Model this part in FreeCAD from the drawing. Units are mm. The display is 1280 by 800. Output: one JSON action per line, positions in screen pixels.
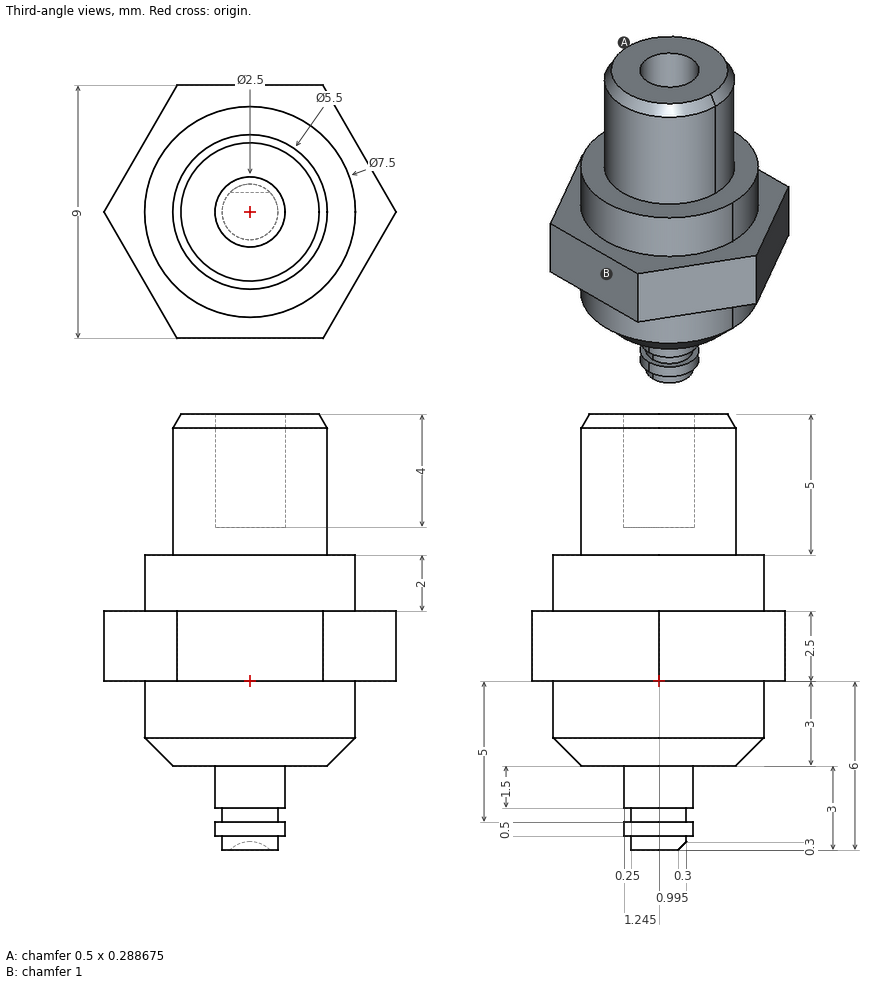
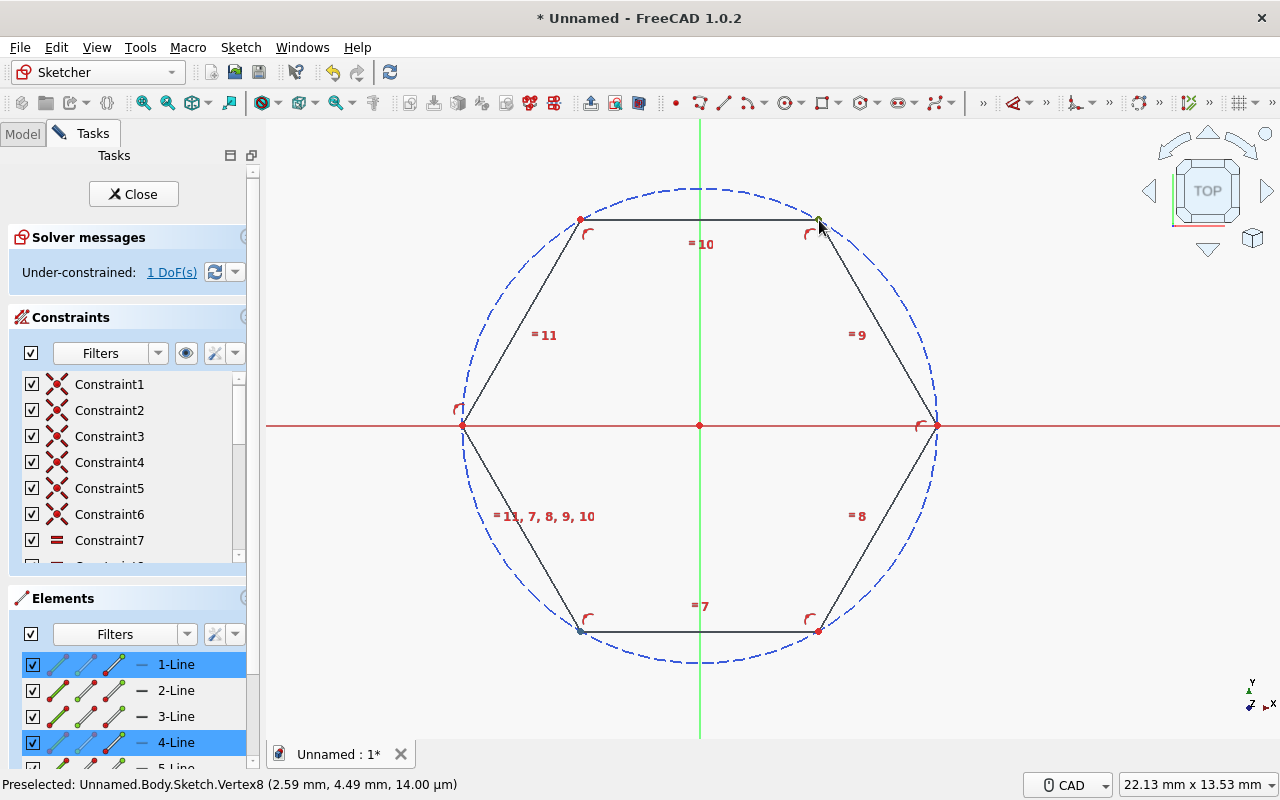
{"action": "key", "text": "i"}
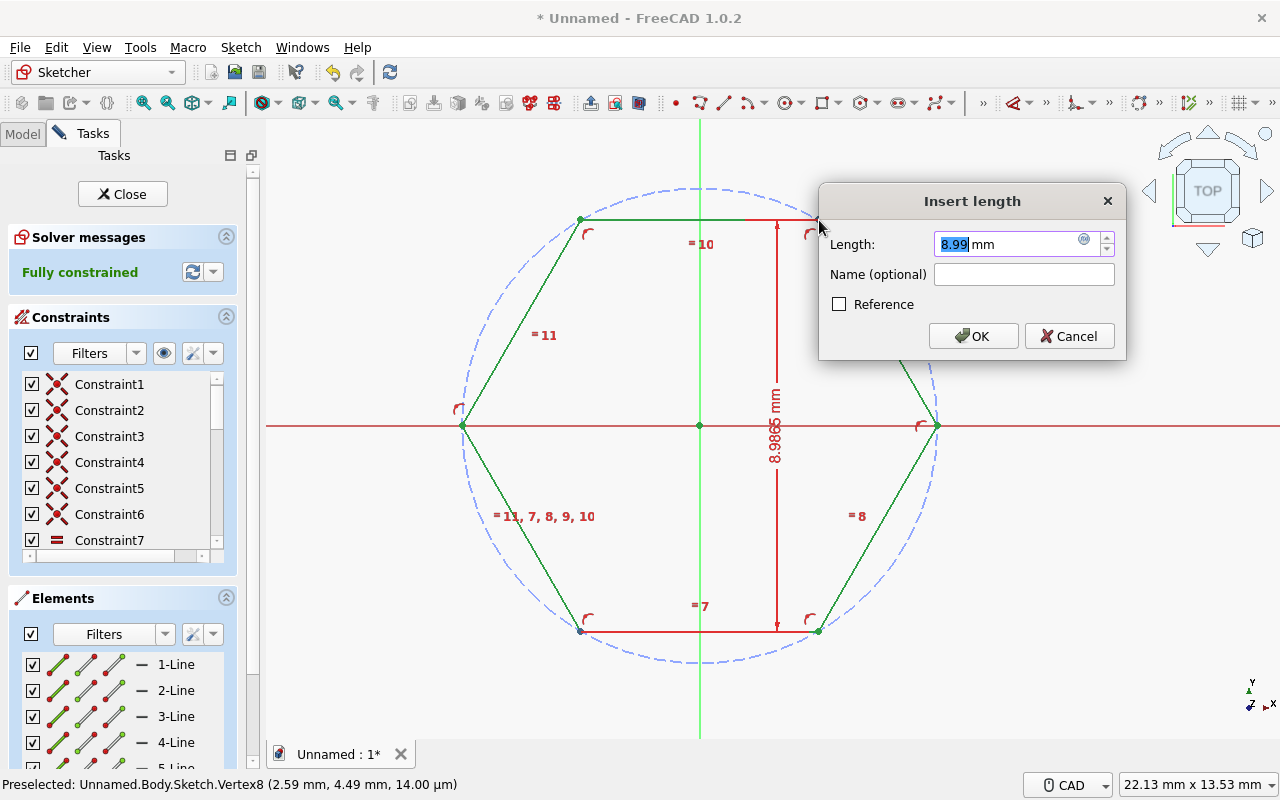
{"action": "type", "text": "9"}
{"action": "key", "text": "Return"}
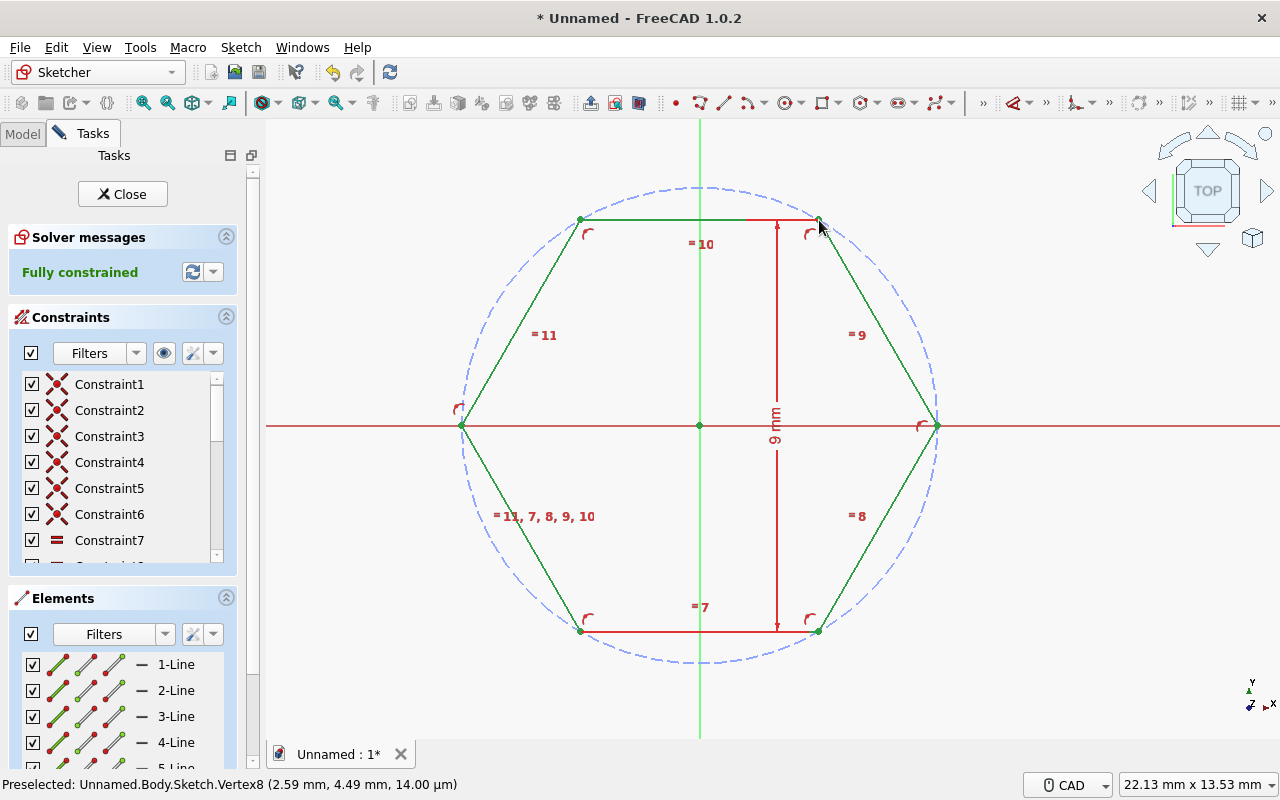
{"action": "left_click", "coordinate": [123, 194]}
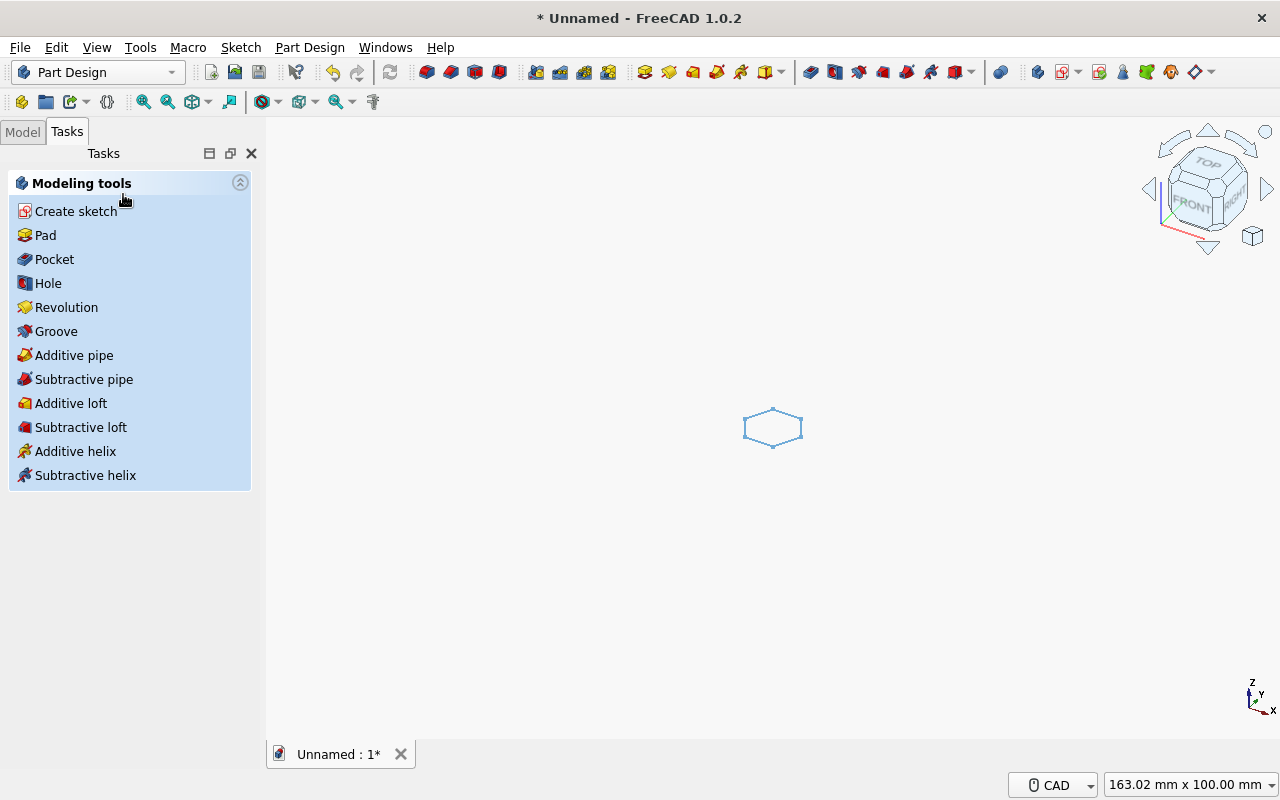
{"action": "left_click", "coordinate": [646, 72]}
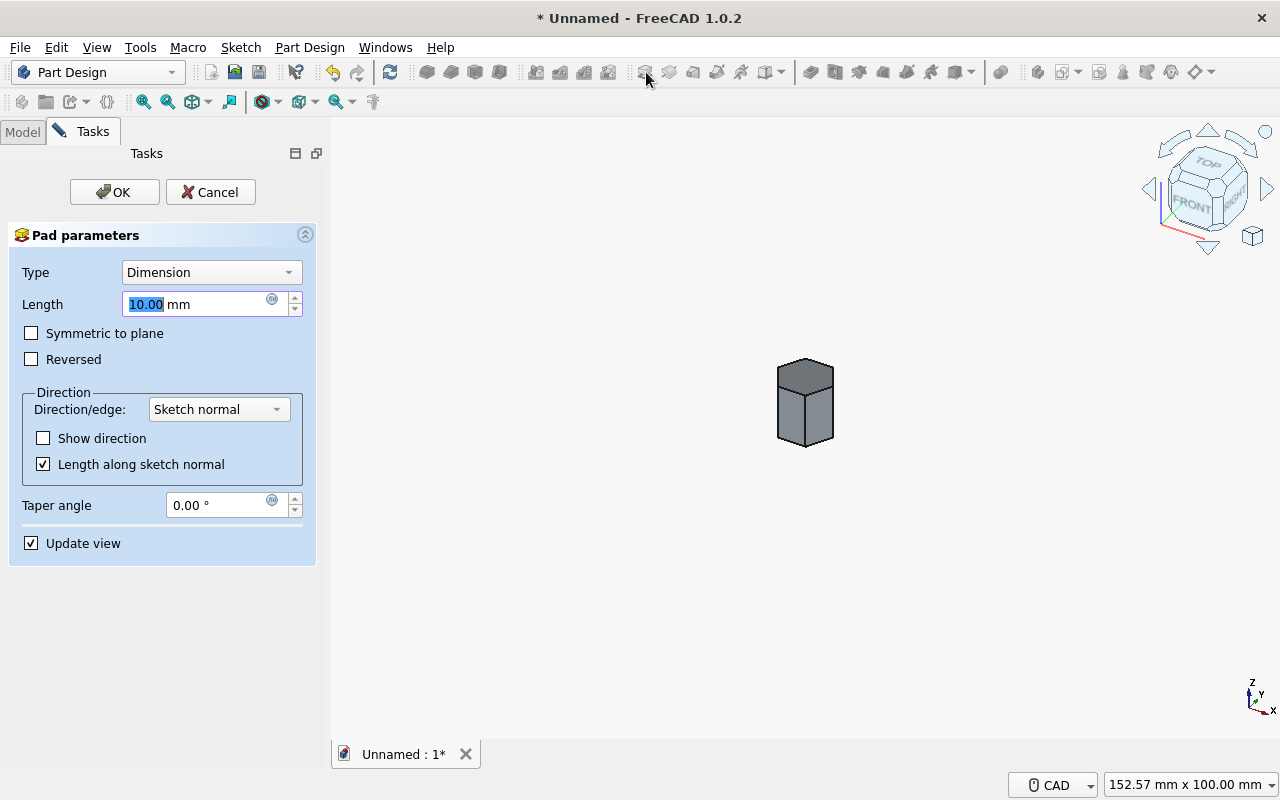
{"action": "type", "text": "2.5"}
{"action": "key", "text": "Tab"}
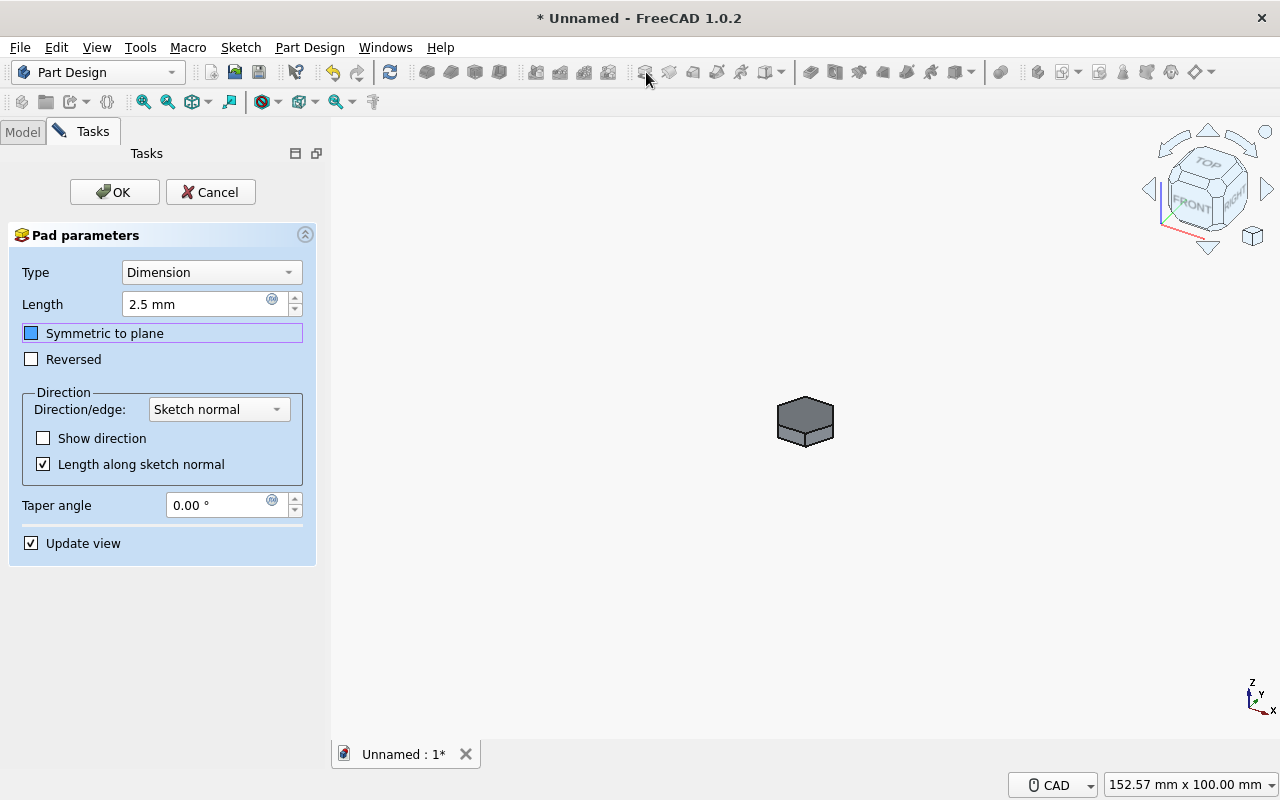
{"action": "left_click", "coordinate": [115, 192]}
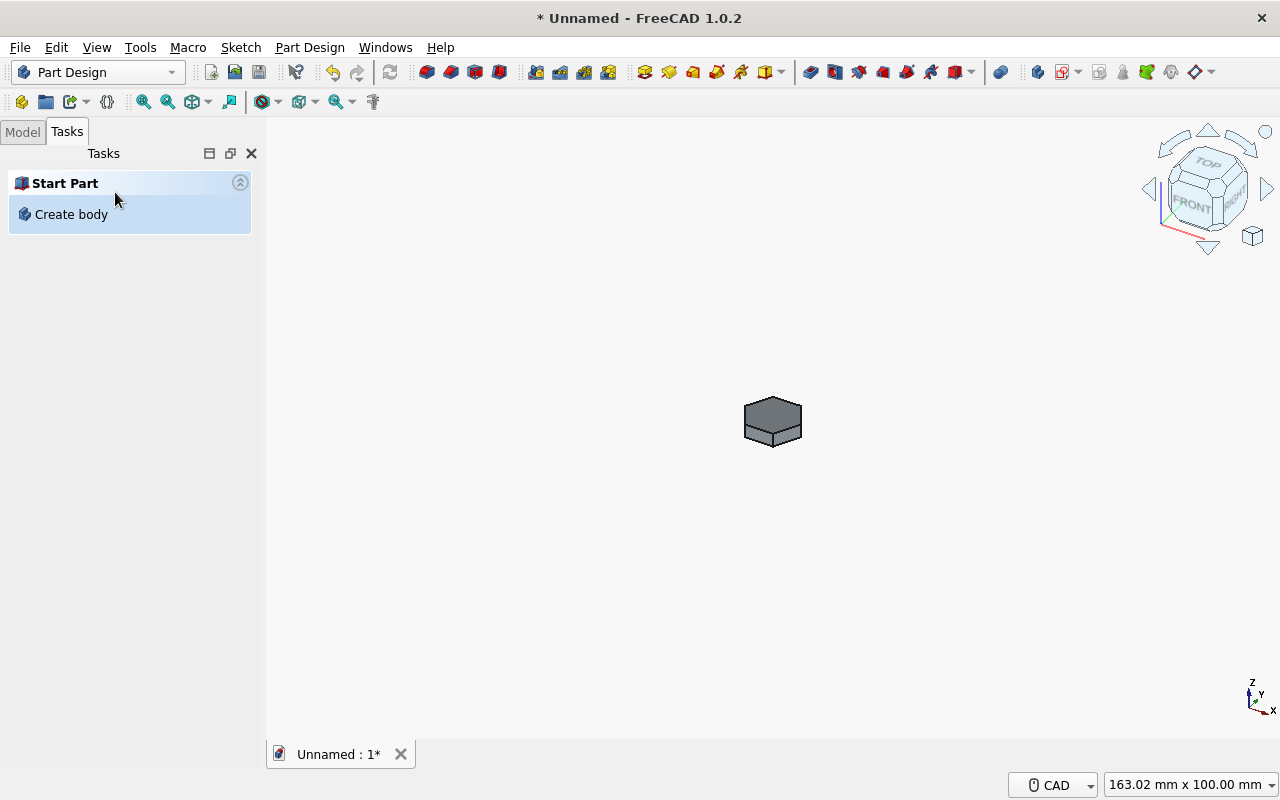
{"action": "key", "text": "v f"}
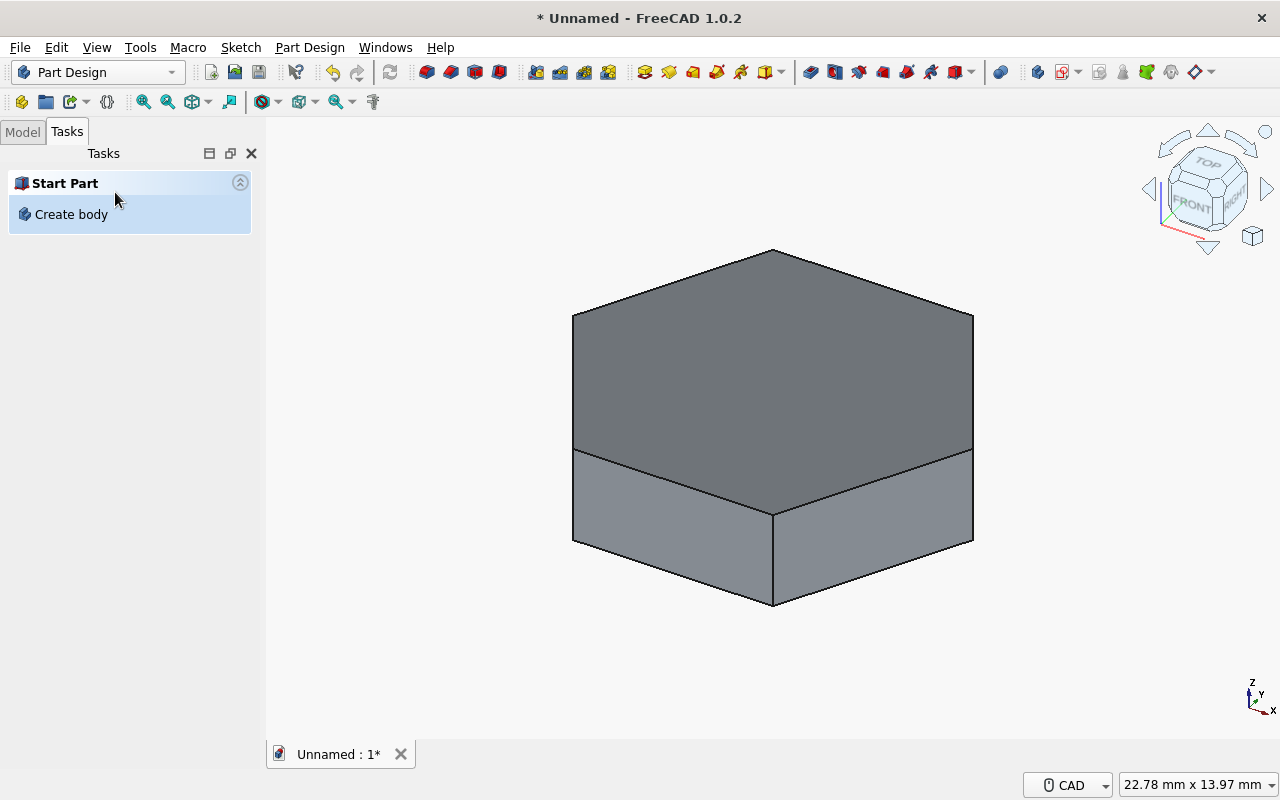
{"action": "left_click", "coordinate": [773, 381]}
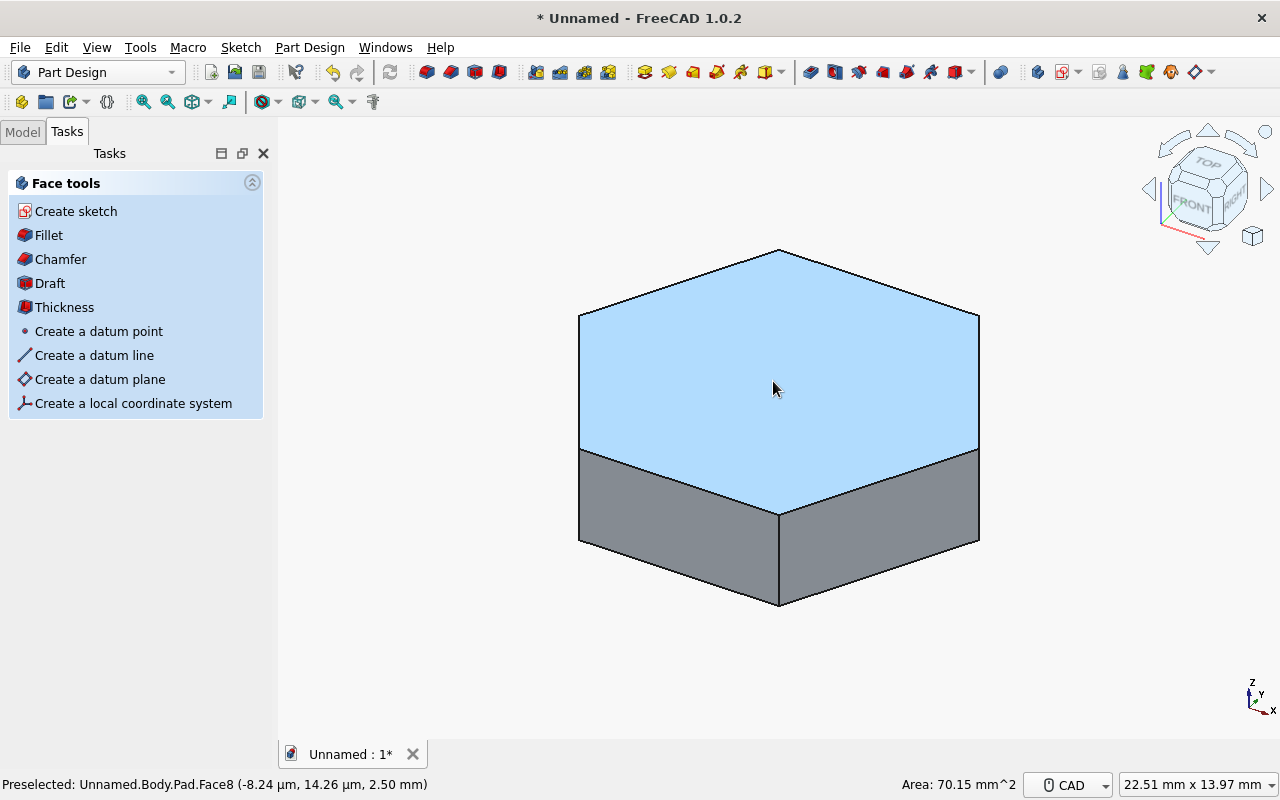
{"action": "left_click", "coordinate": [1062, 72]}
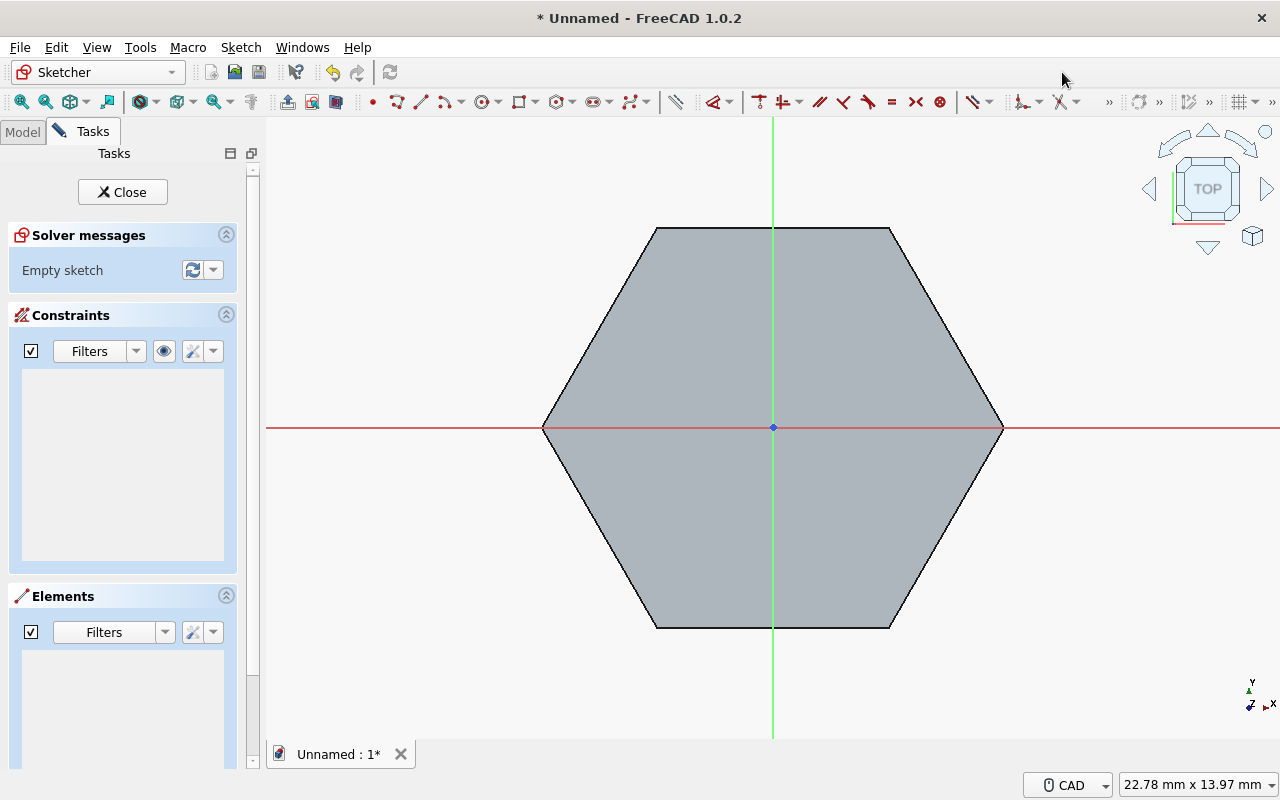
{"action": "key", "text": "g c"}